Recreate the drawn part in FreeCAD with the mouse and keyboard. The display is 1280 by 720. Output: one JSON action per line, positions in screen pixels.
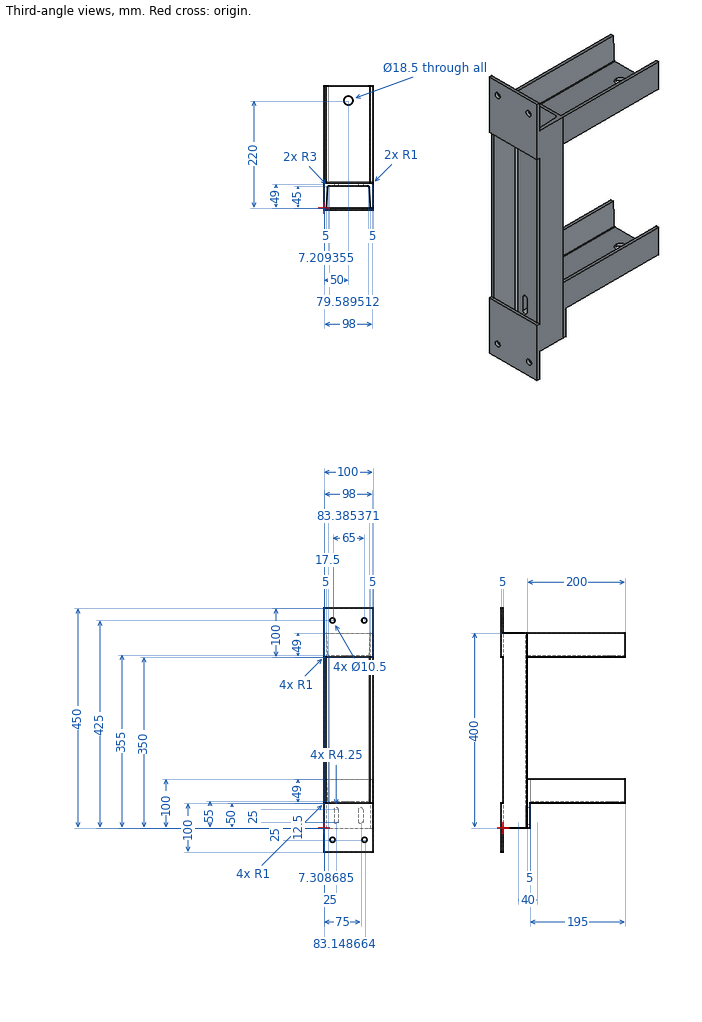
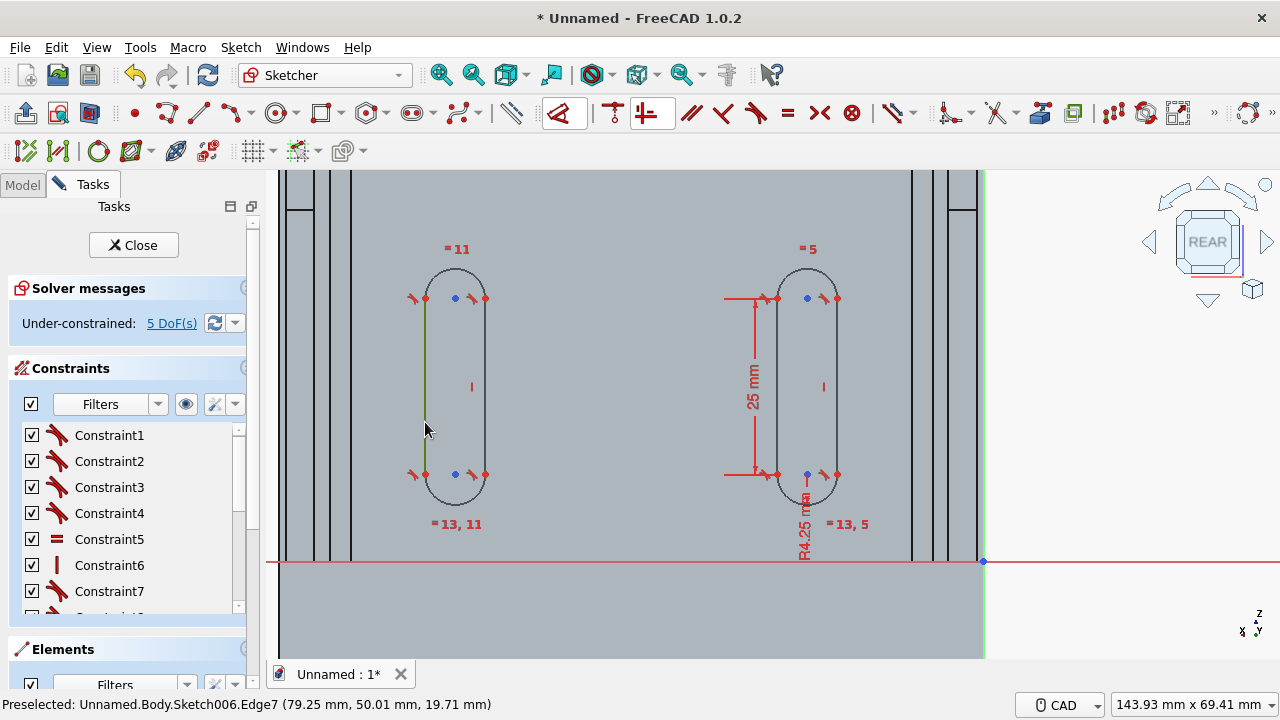
{"action": "key", "text": "i"}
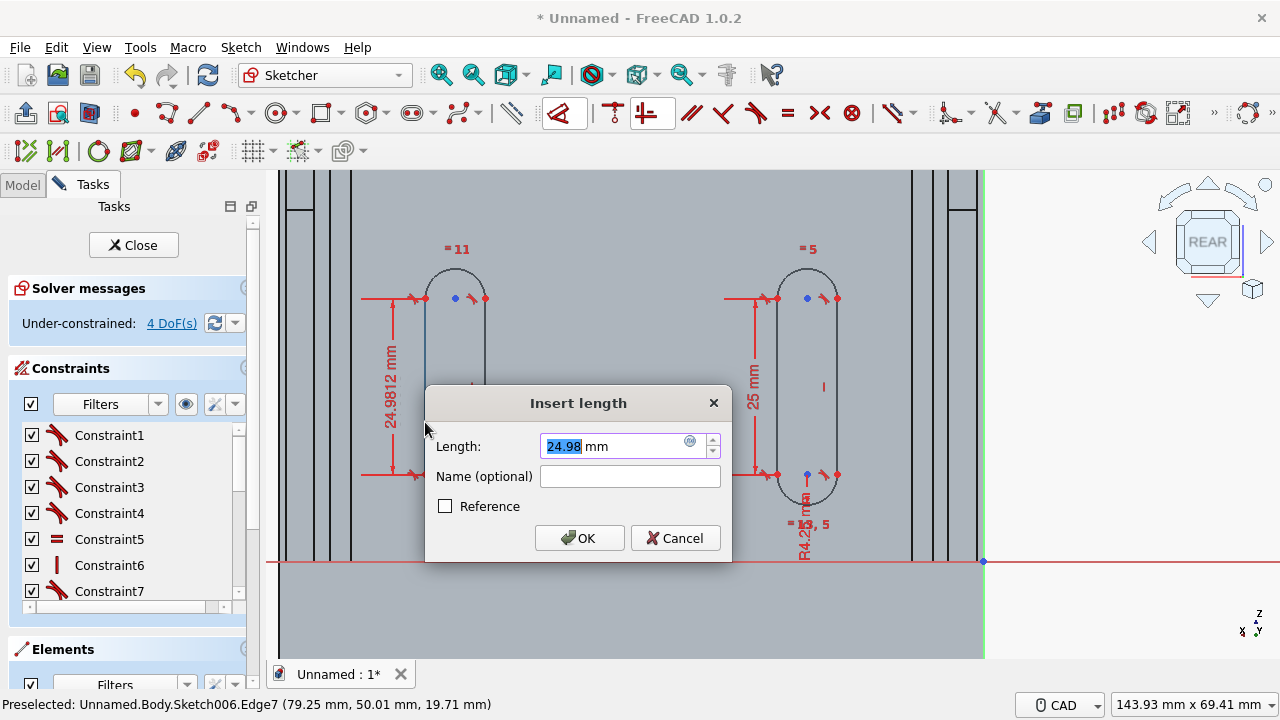
{"action": "type", "text": "25"}
{"action": "key", "text": "Return"}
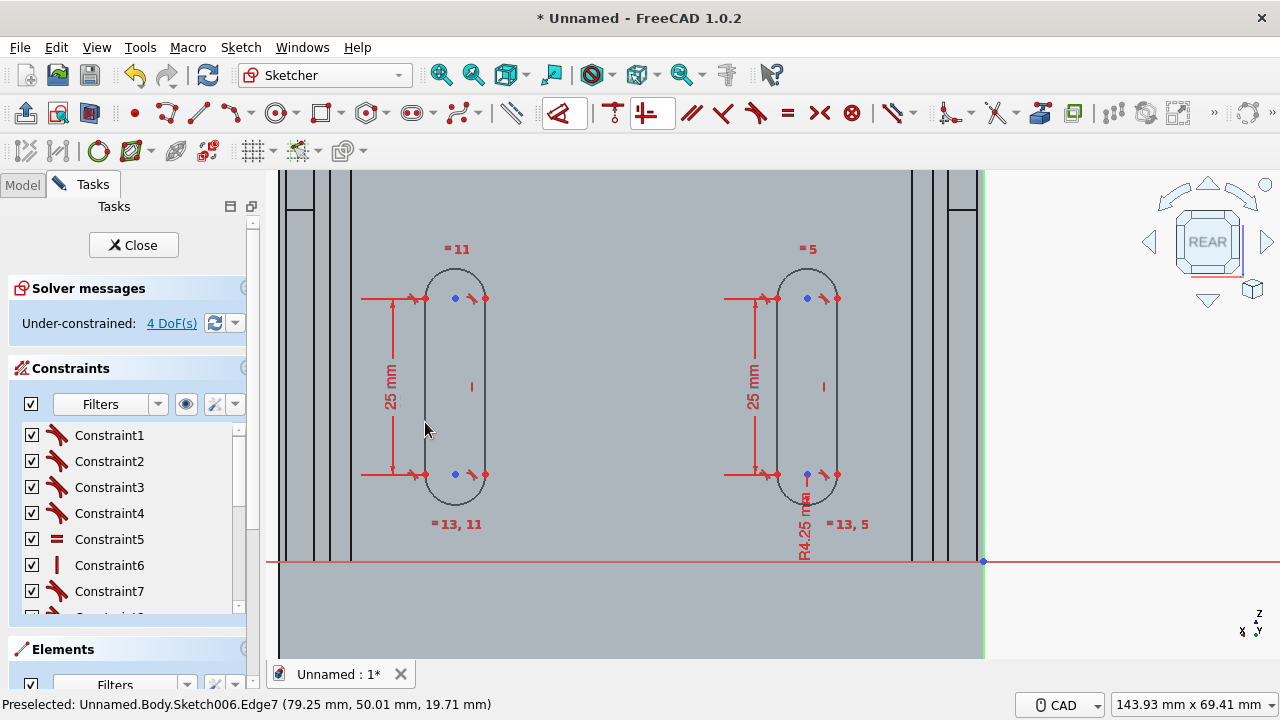
{"action": "left_click", "coordinate": [807, 475]}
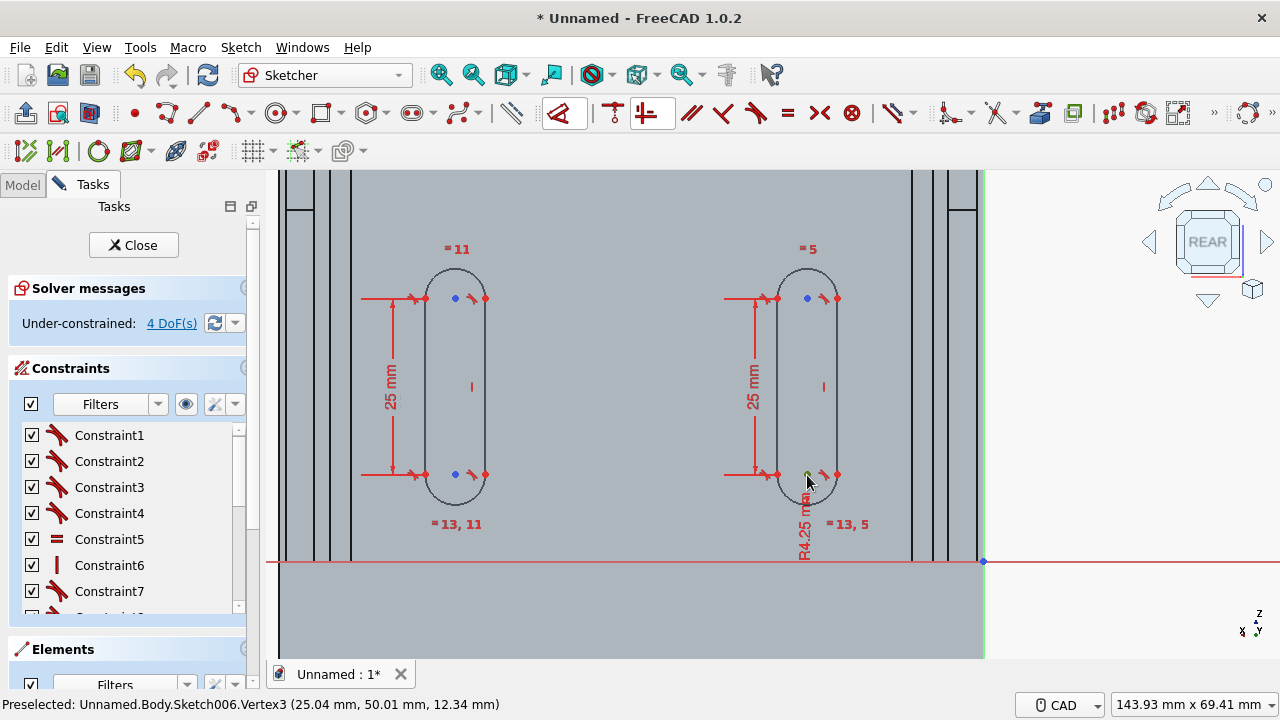
{"action": "key", "text": "l"}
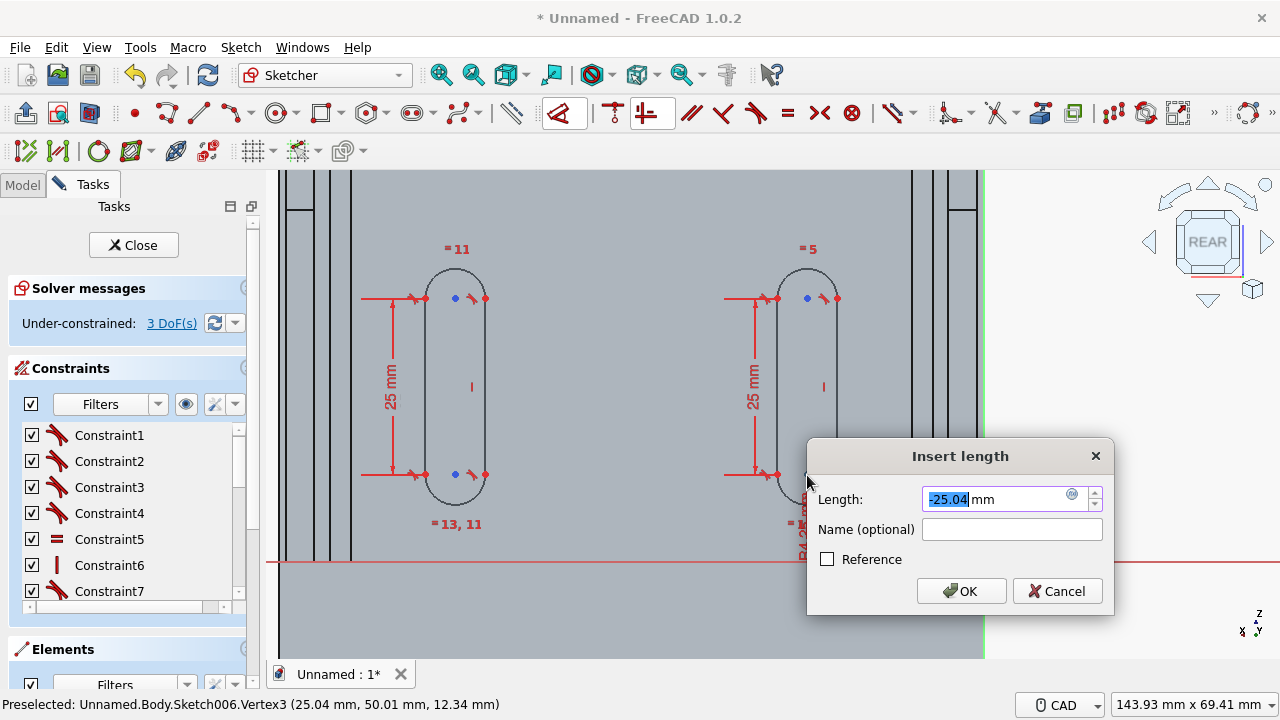
{"action": "type", "text": "-25"}
{"action": "key", "text": "Return"}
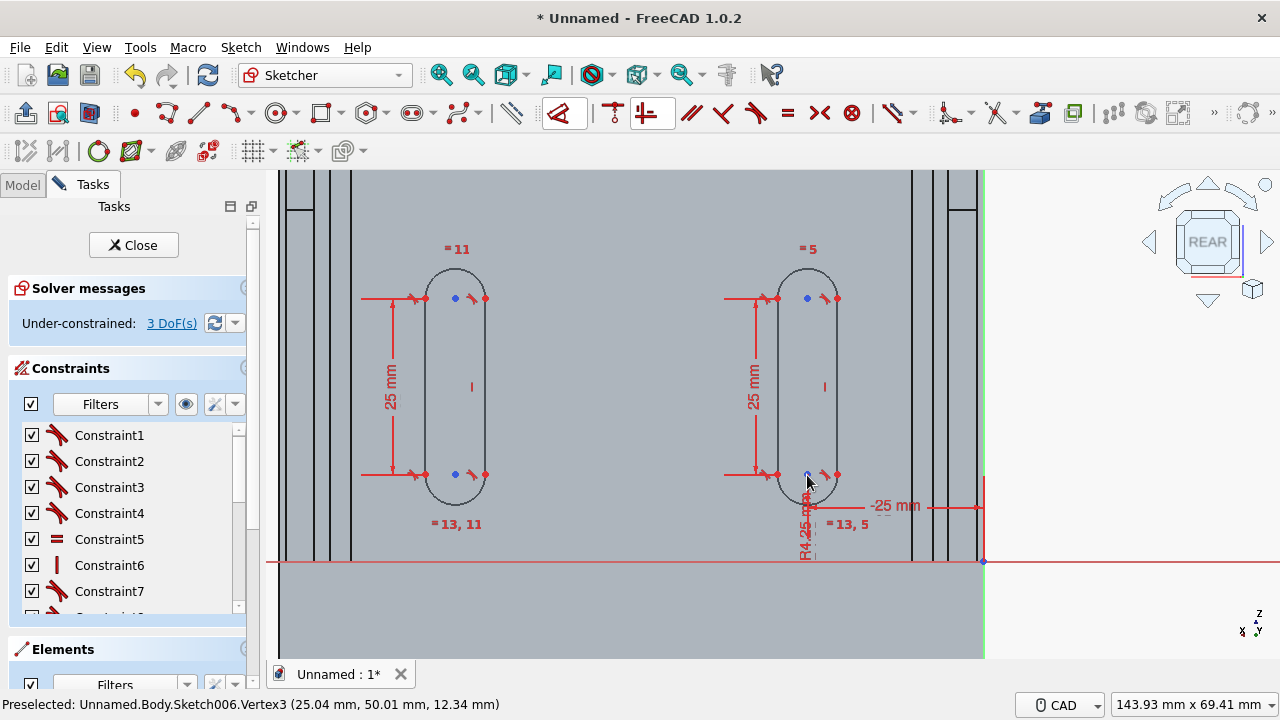
{"action": "left_click", "coordinate": [455, 475]}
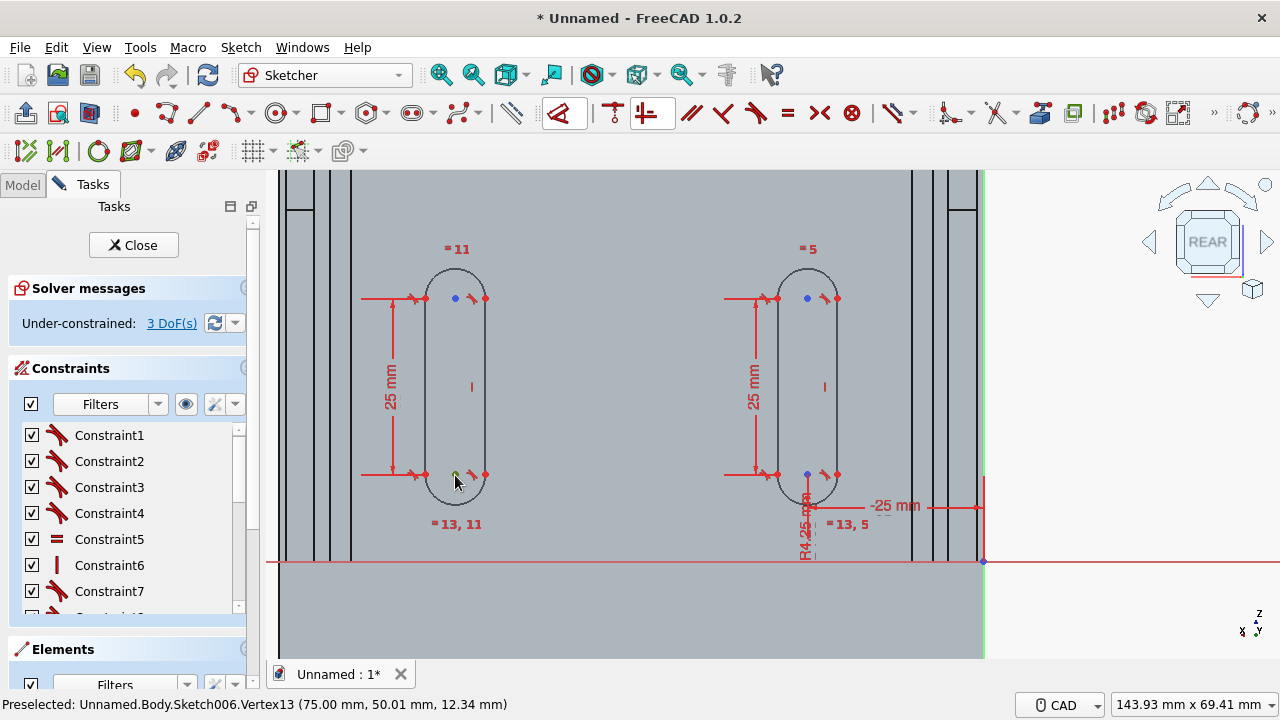
{"action": "left_click", "coordinate": [582, 114]}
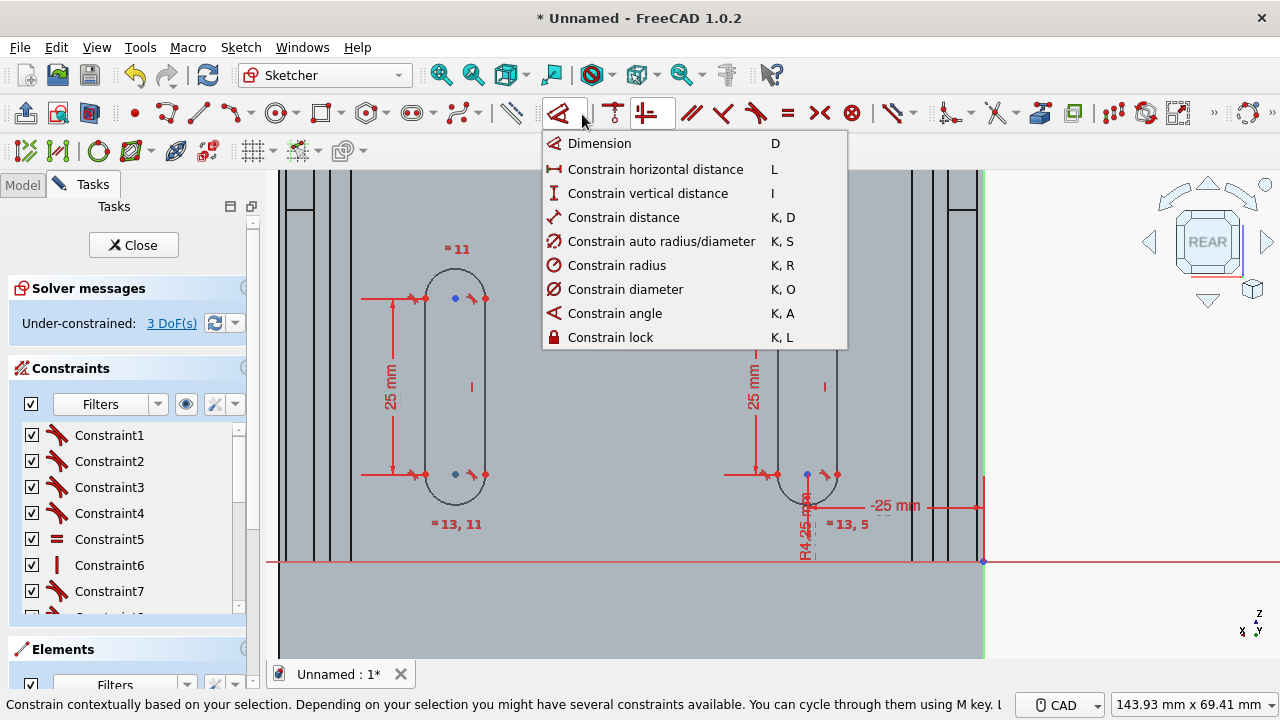
{"action": "left_click", "coordinate": [695, 169]}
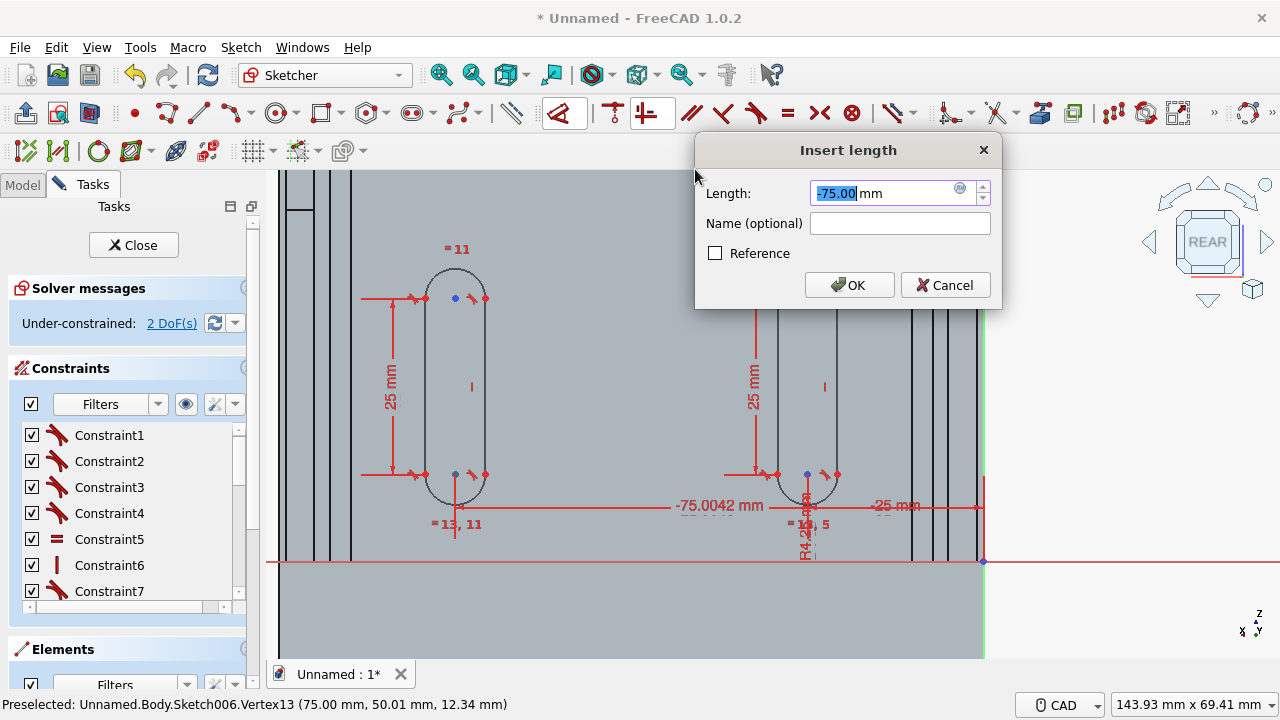
{"action": "type", "text": "-75"}
{"action": "key", "text": "Return"}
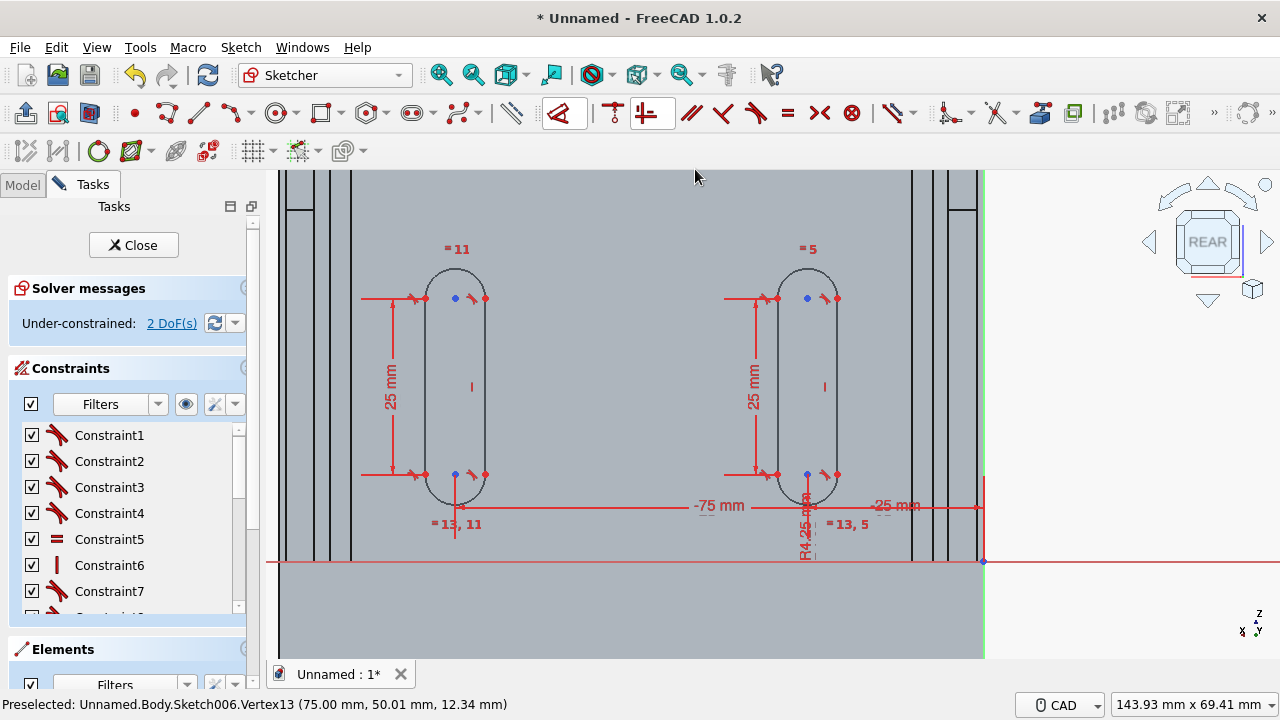
{"action": "left_click", "coordinate": [778, 475]}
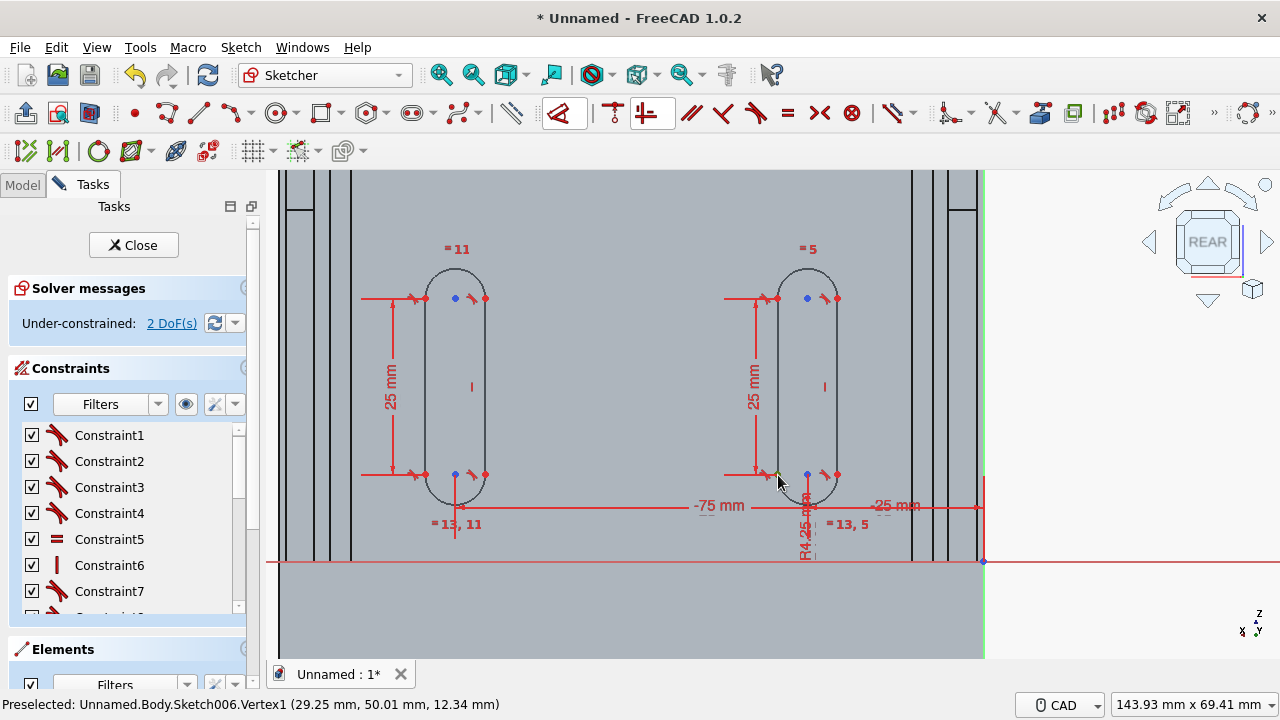
{"action": "left_click", "coordinate": [582, 114]}